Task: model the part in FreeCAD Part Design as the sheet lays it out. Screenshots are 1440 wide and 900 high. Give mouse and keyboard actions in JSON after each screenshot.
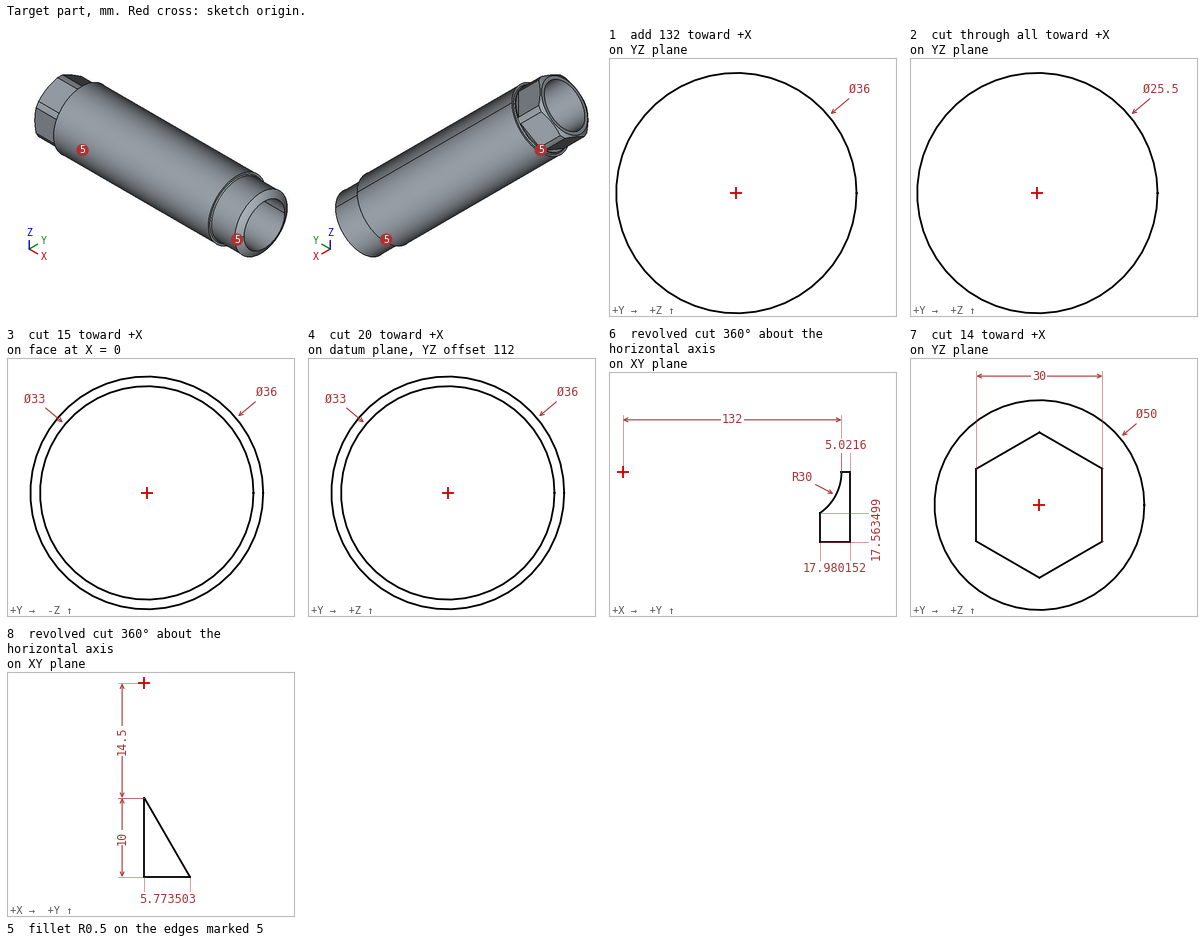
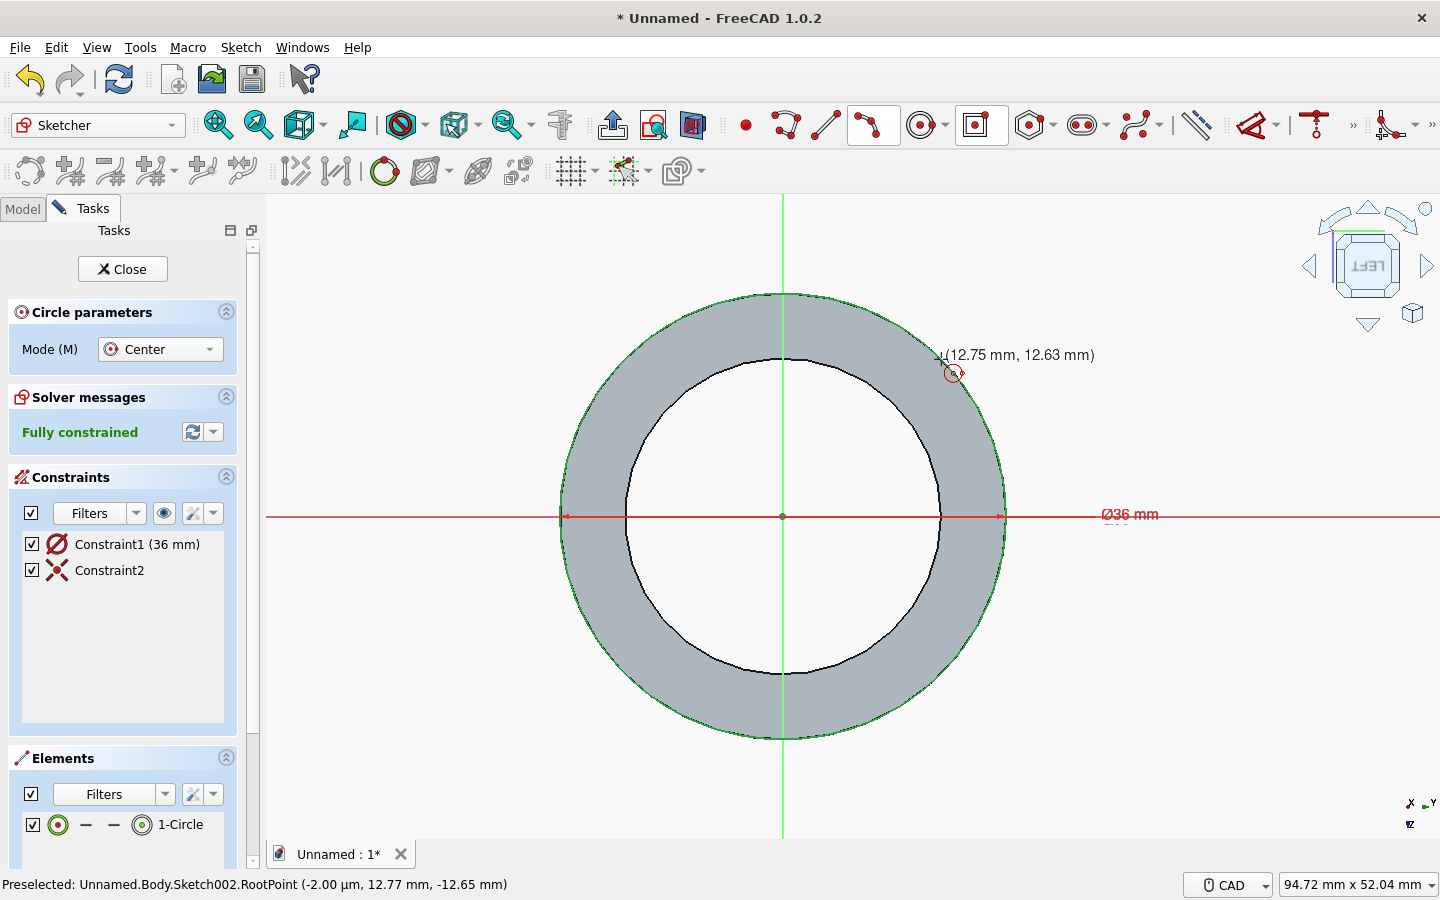
{"action": "left_click", "coordinate": [783, 516]}
{"action": "mouse_move", "coordinate": [928, 372]}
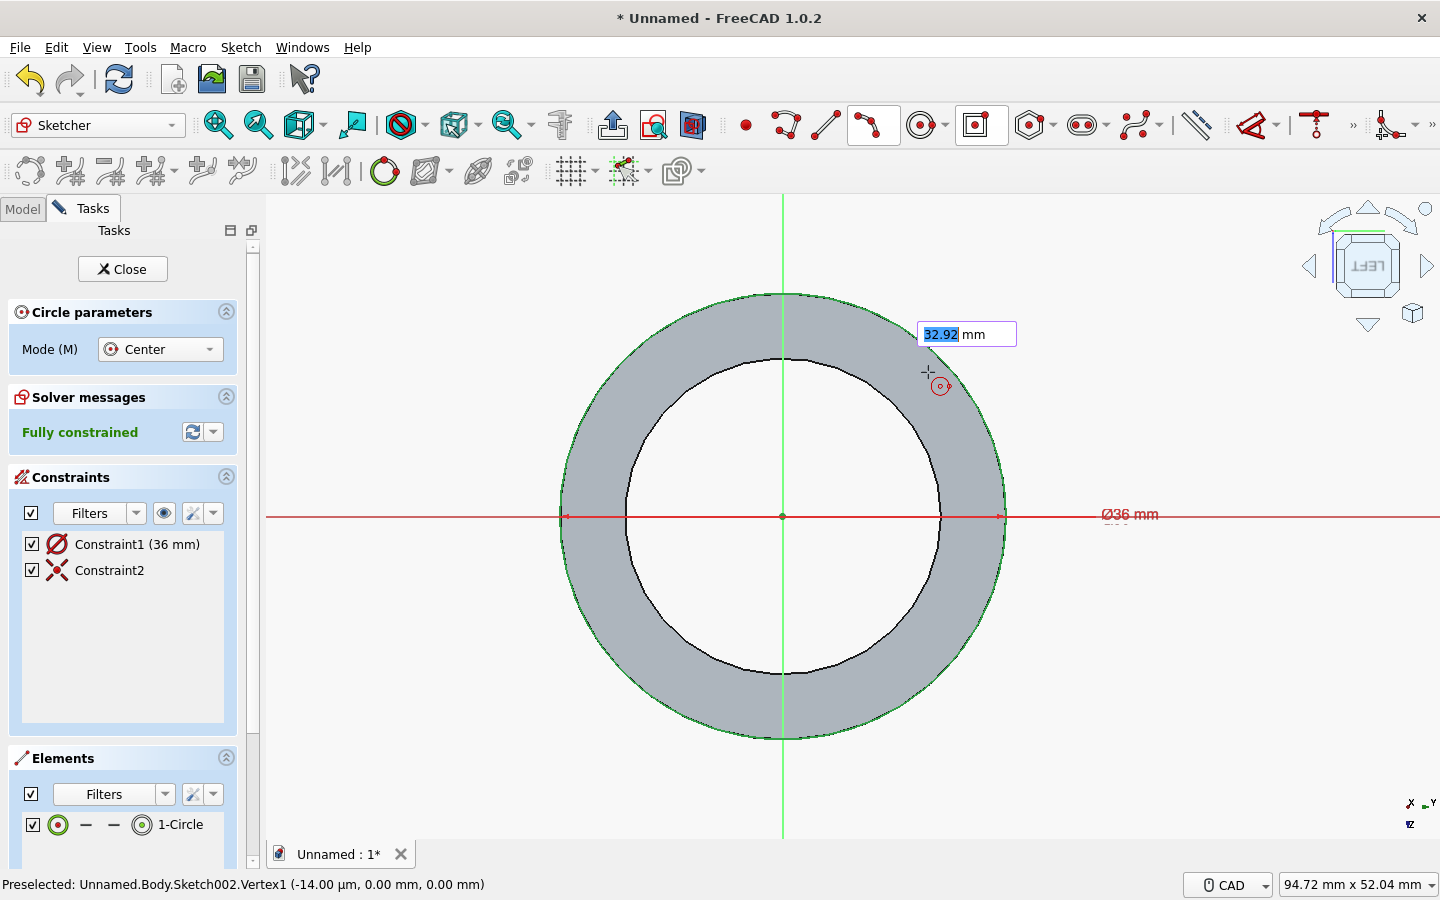
{"action": "type", "text": "33"}
{"action": "key", "text": "Return"}
{"action": "key", "text": "Escape"}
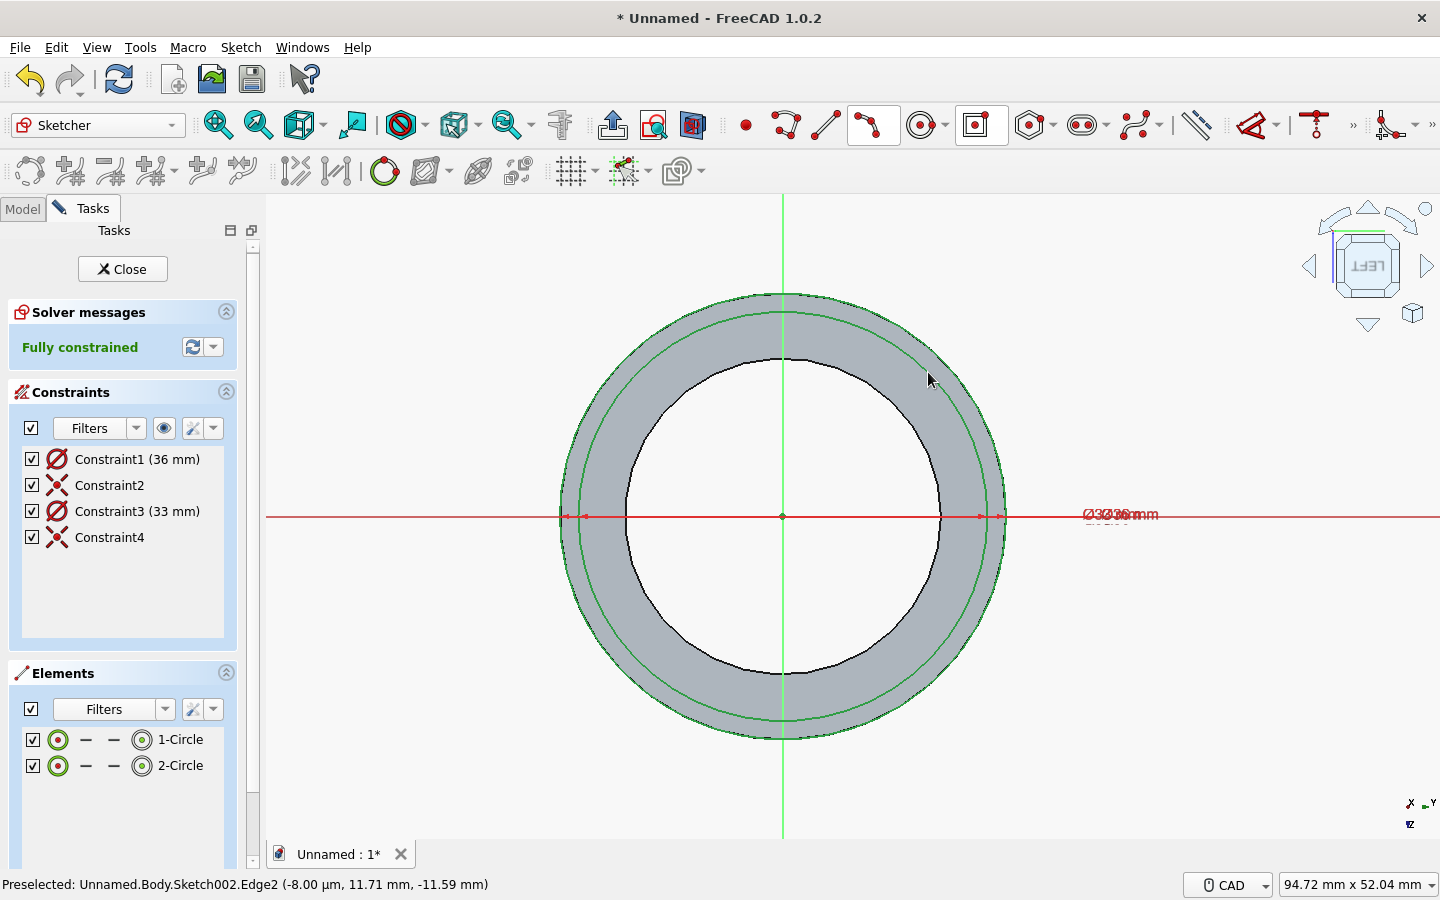
{"action": "left_click", "coordinate": [123, 269]}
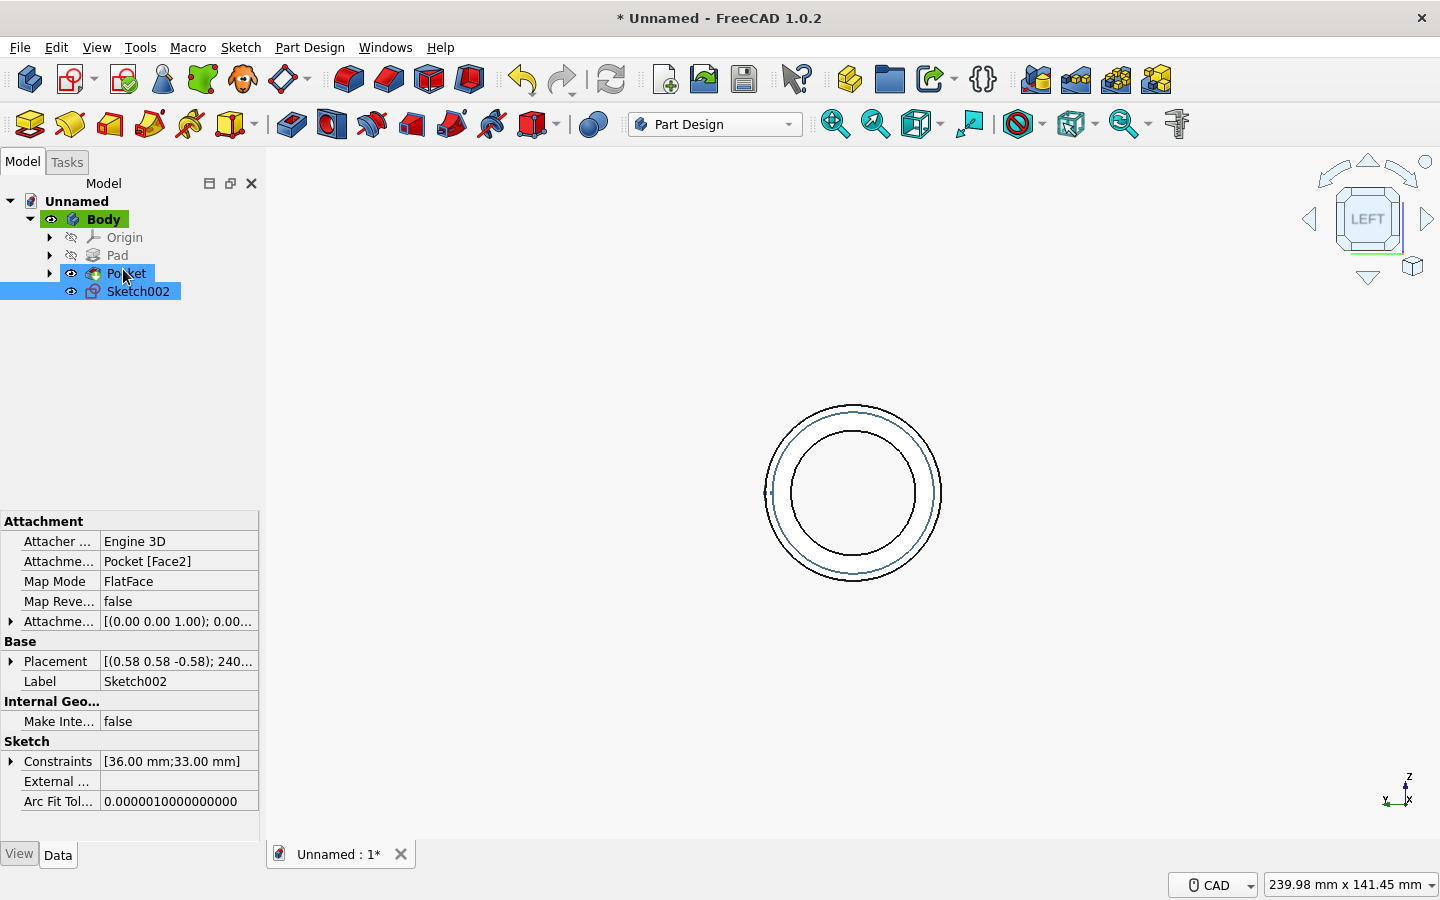
{"action": "left_click", "coordinate": [292, 124]}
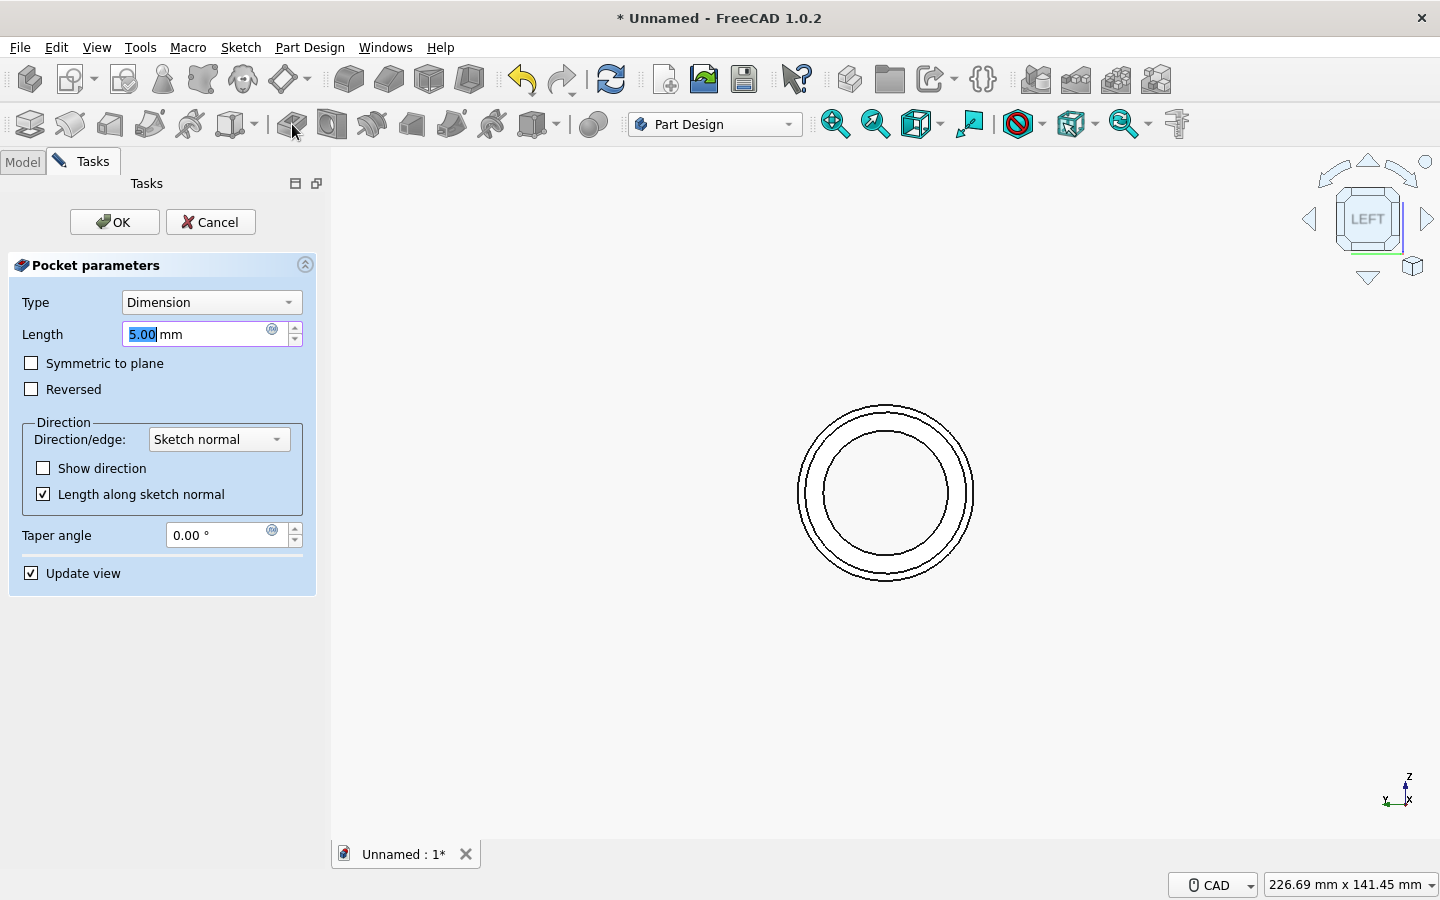
{"action": "type", "text": "15"}
{"action": "key", "text": "Tab"}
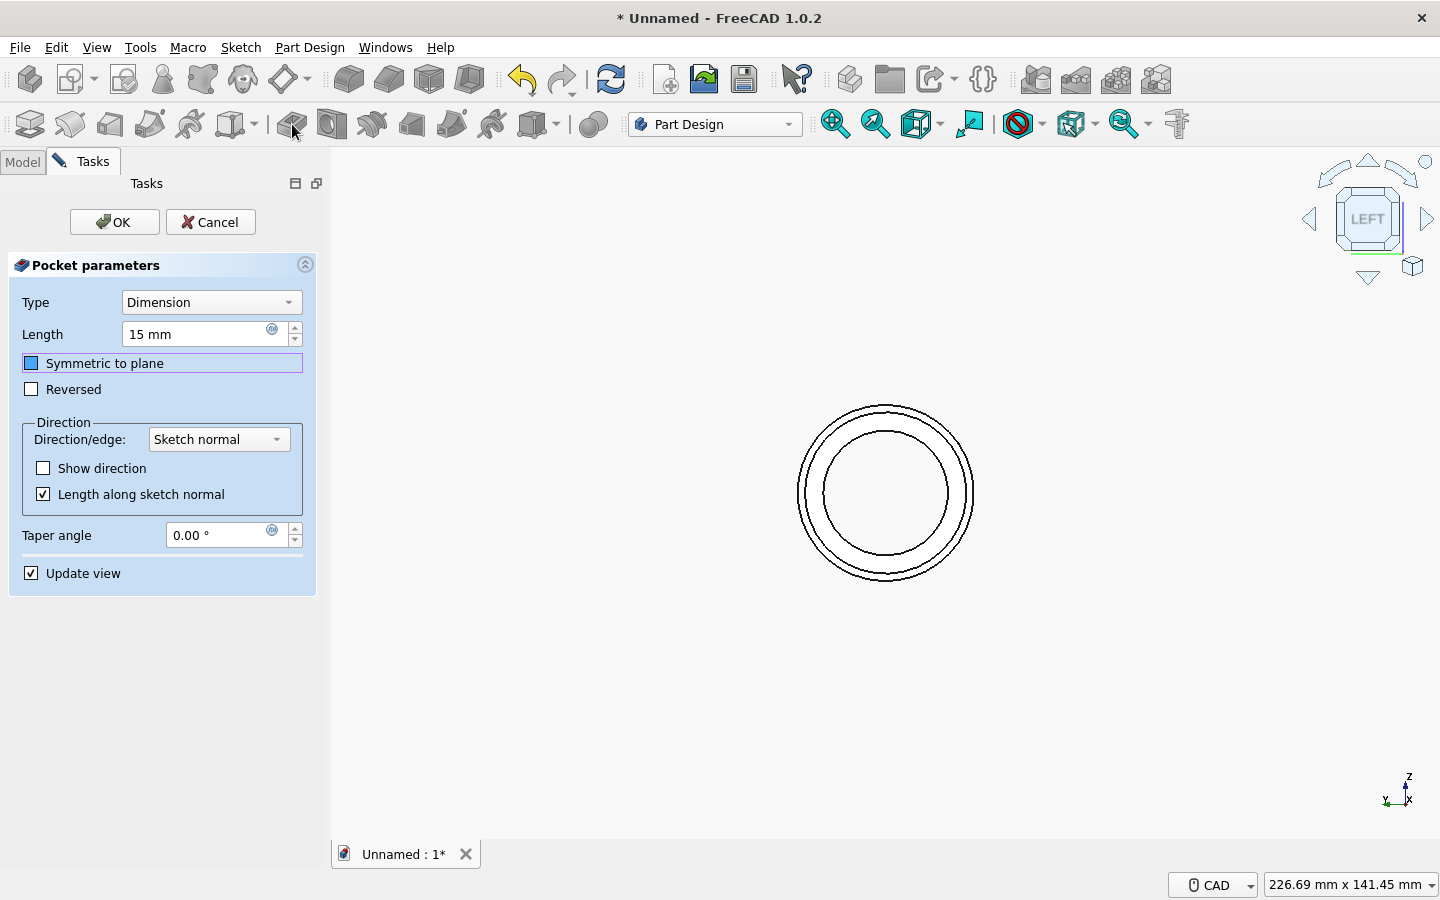
{"action": "left_click", "coordinate": [115, 222]}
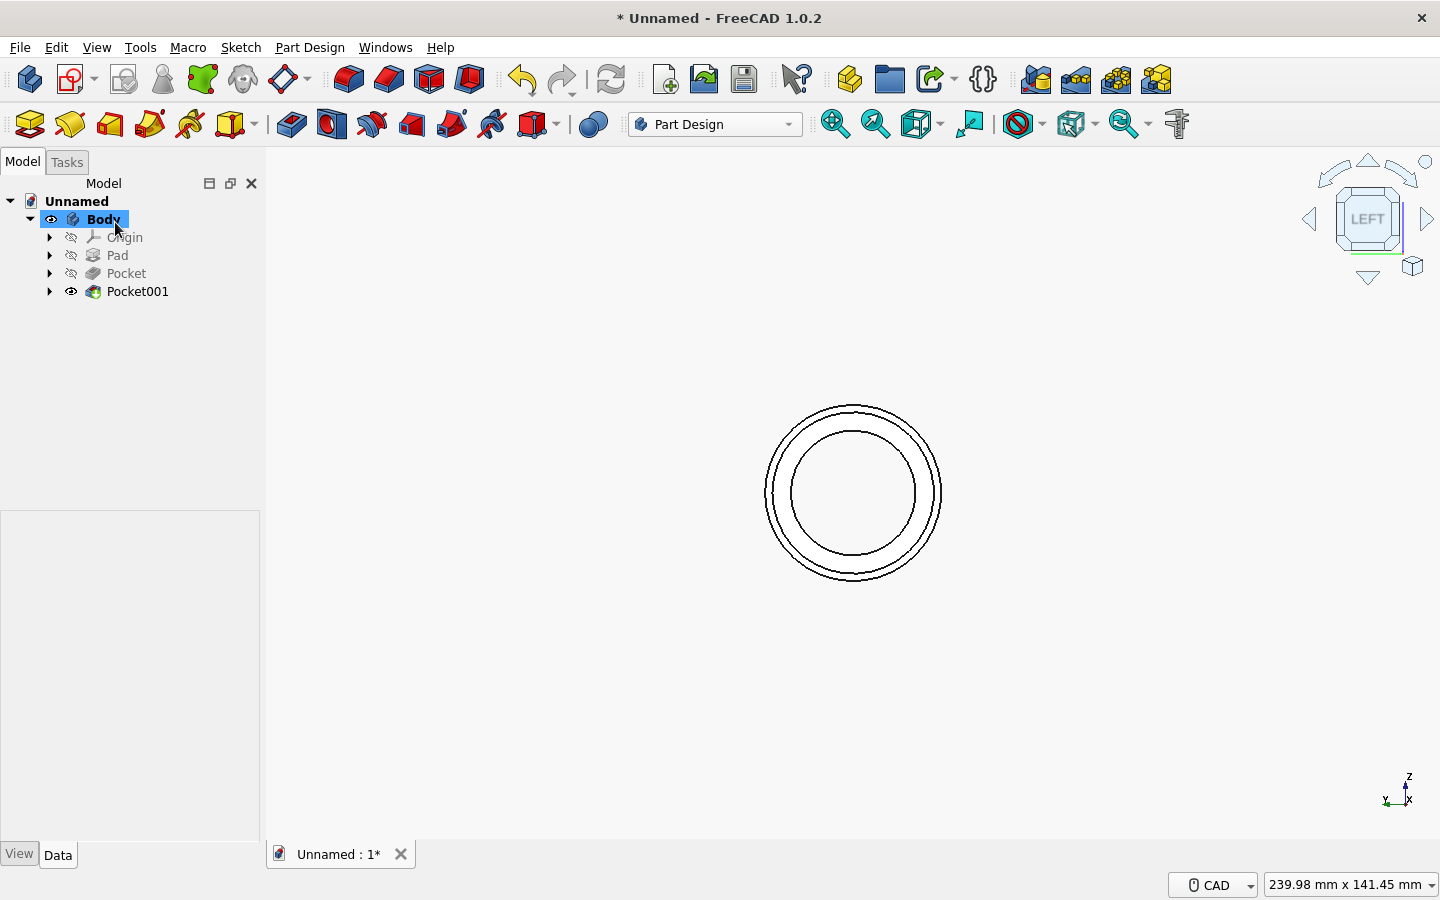
{"action": "key", "text": "v f"}